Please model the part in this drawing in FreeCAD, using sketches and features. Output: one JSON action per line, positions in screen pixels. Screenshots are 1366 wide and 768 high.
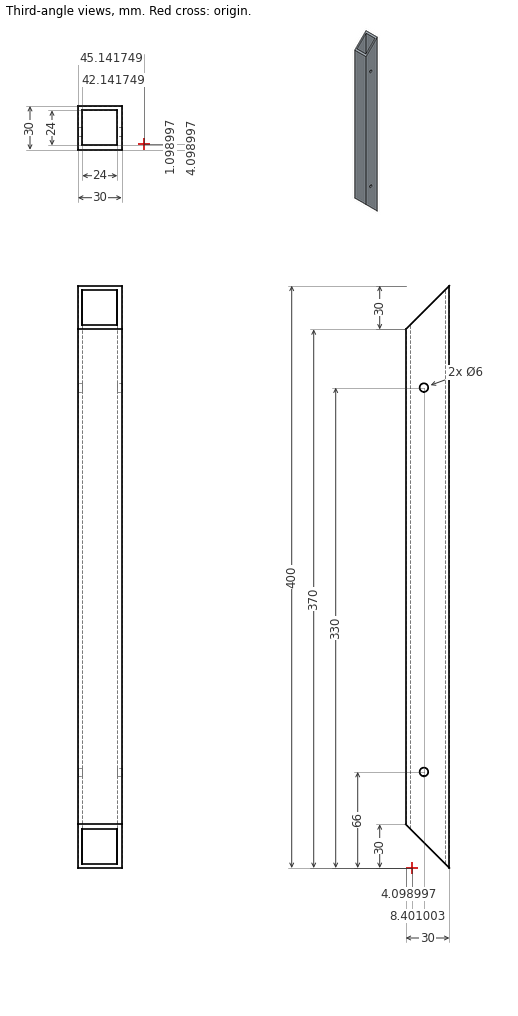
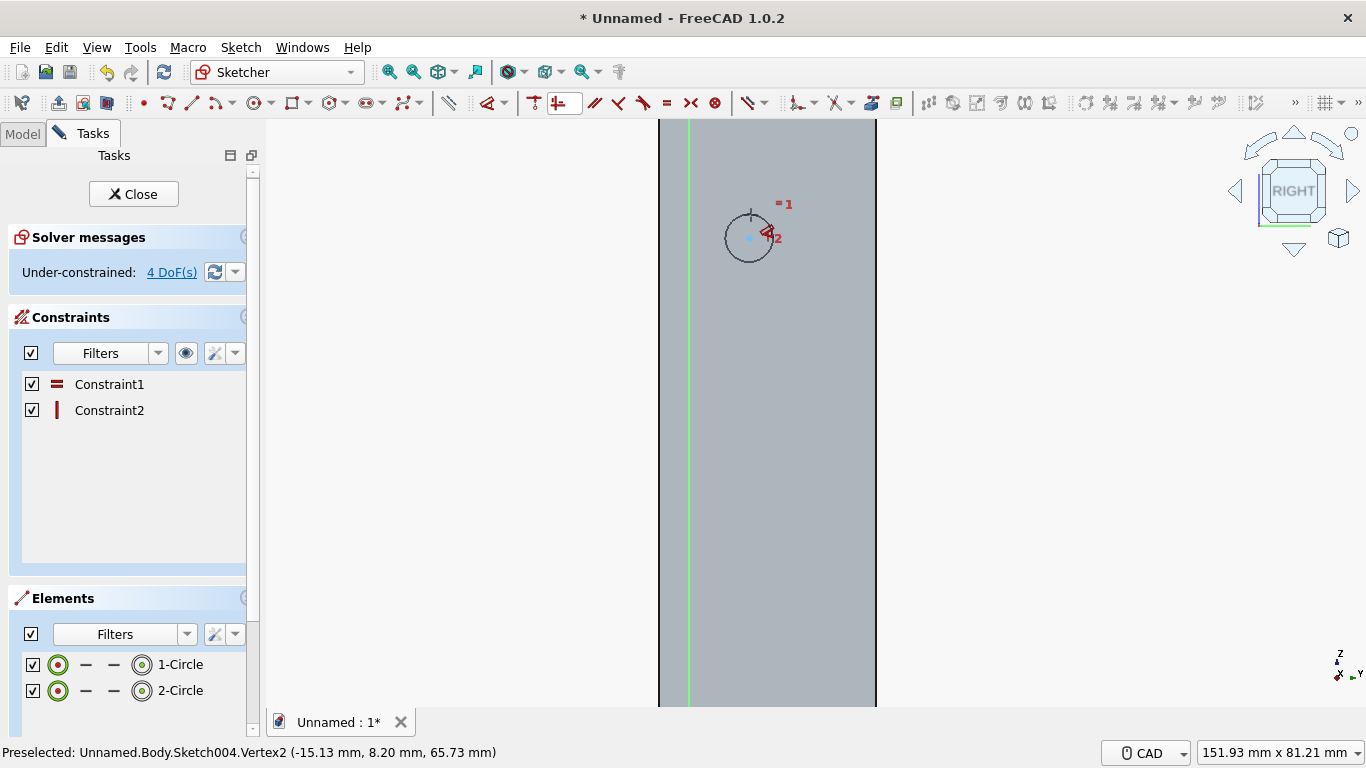
{"action": "left_click", "coordinate": [750, 214]}
{"action": "left_click", "coordinate": [751, 182]}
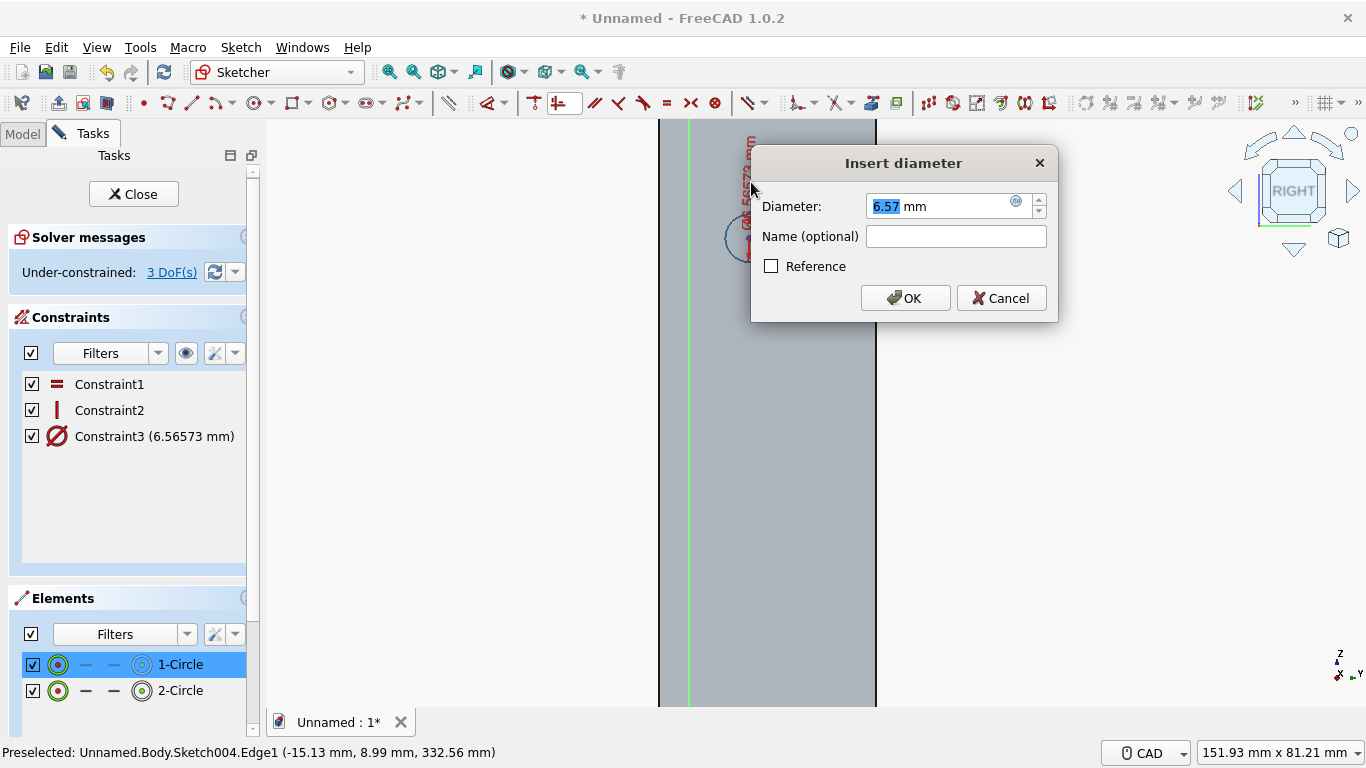
{"action": "type", "text": "6"}
{"action": "key", "text": "Return"}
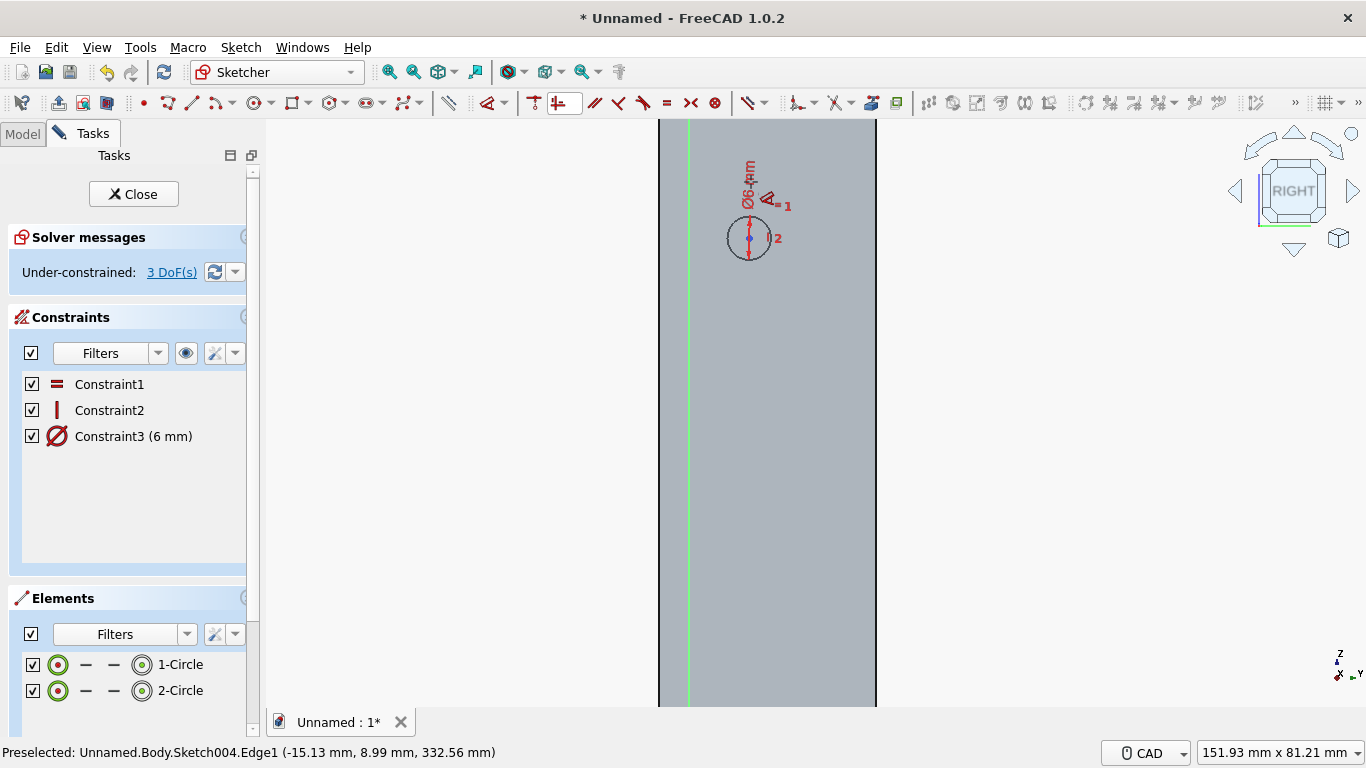
{"action": "scroll", "coordinate": [751, 214], "scroll_direction": "down", "scroll_amount": 9}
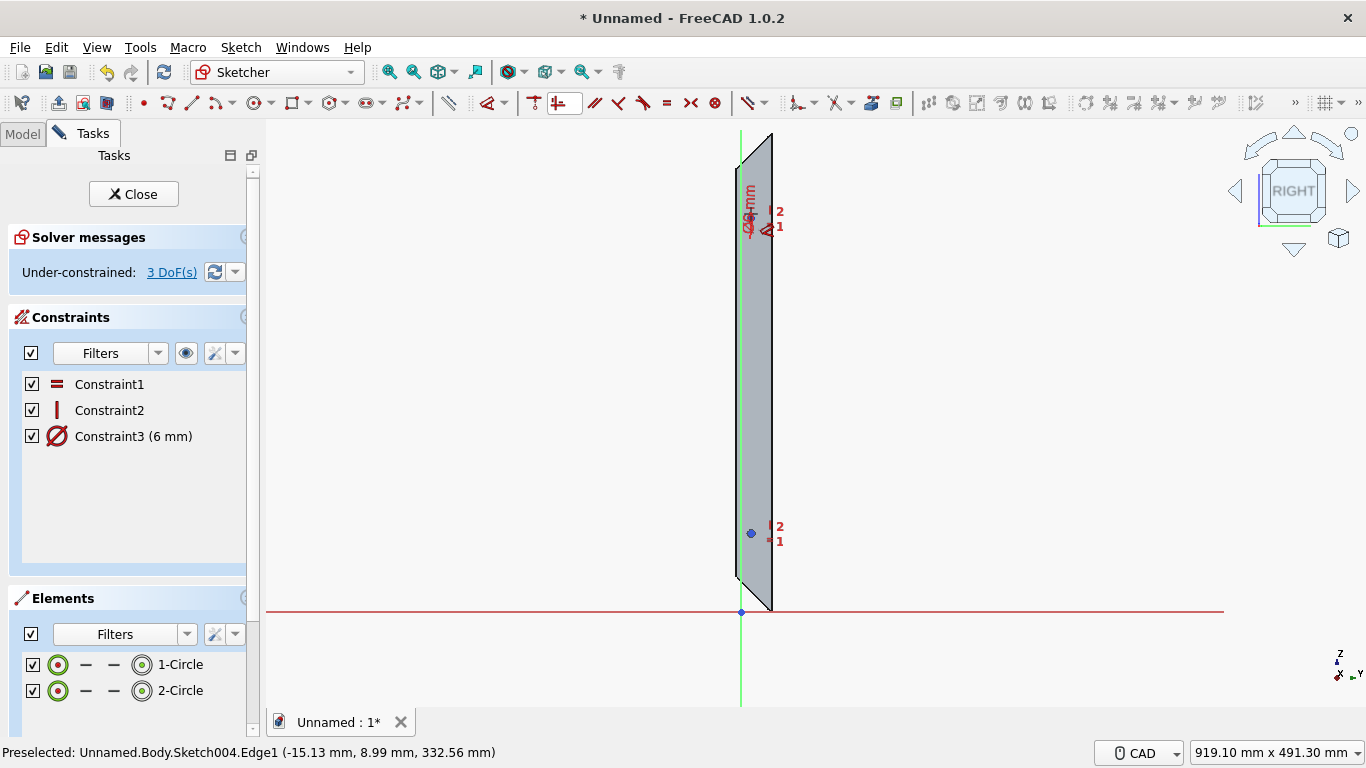
{"action": "left_click", "coordinate": [751, 534]}
{"action": "left_click", "coordinate": [707, 573]}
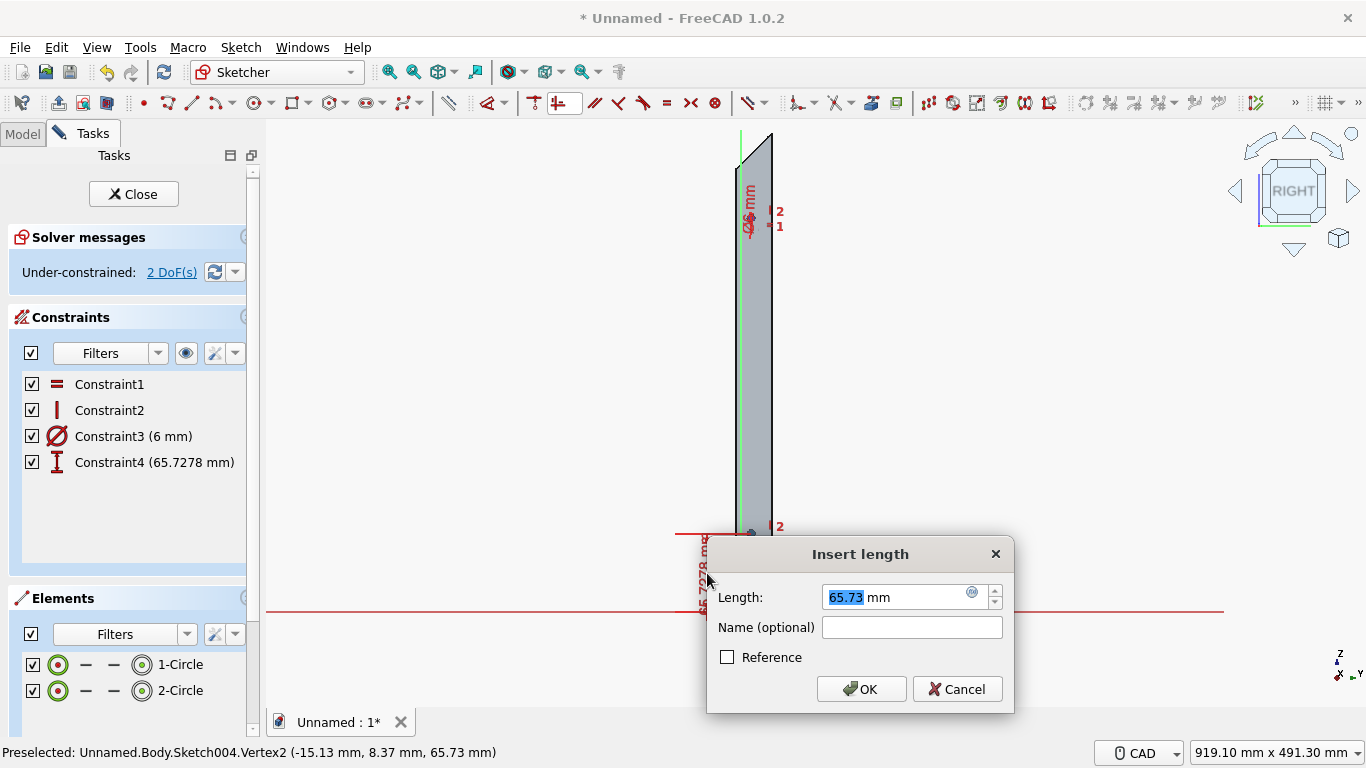
{"action": "type", "text": "66"}
{"action": "key", "text": "Return"}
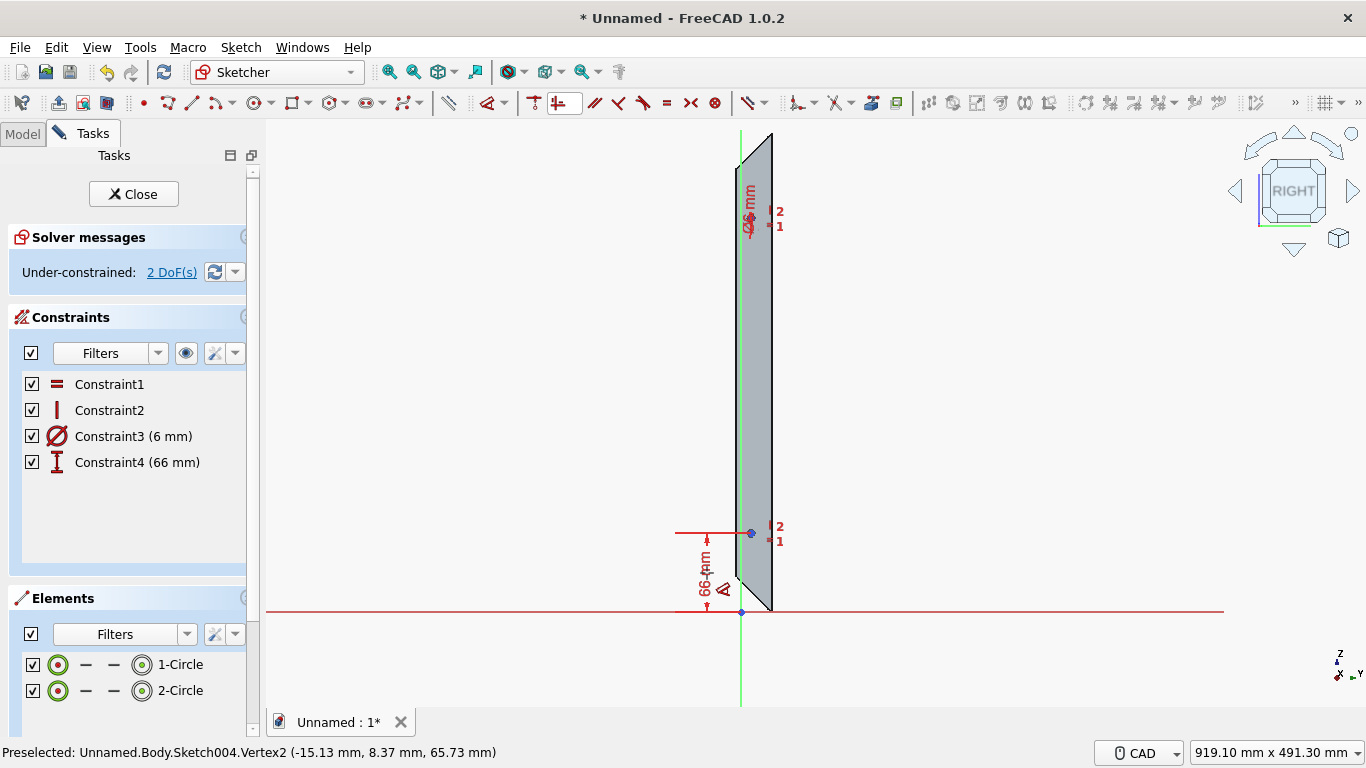
{"action": "left_click", "coordinate": [751, 218]}
{"action": "left_click", "coordinate": [707, 415]}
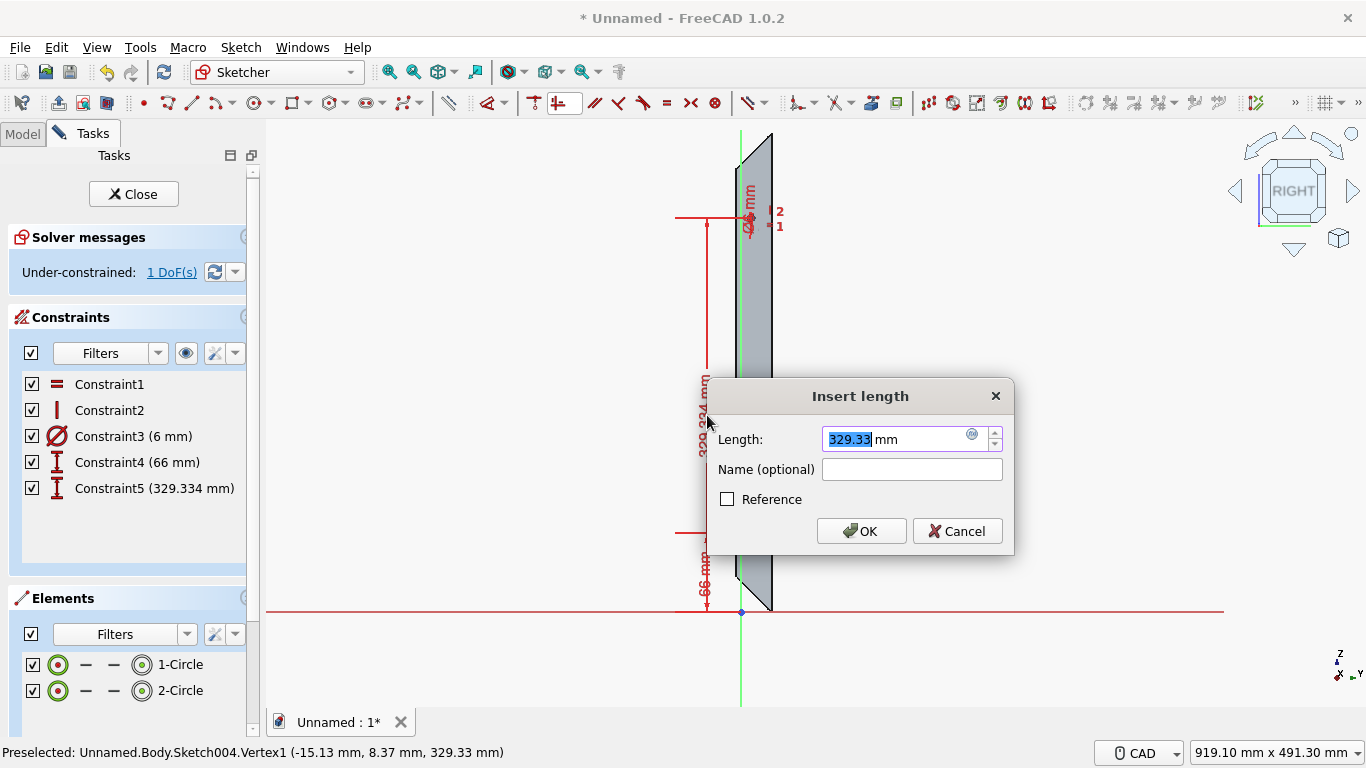
{"action": "type", "text": "330"}
{"action": "key", "text": "Return"}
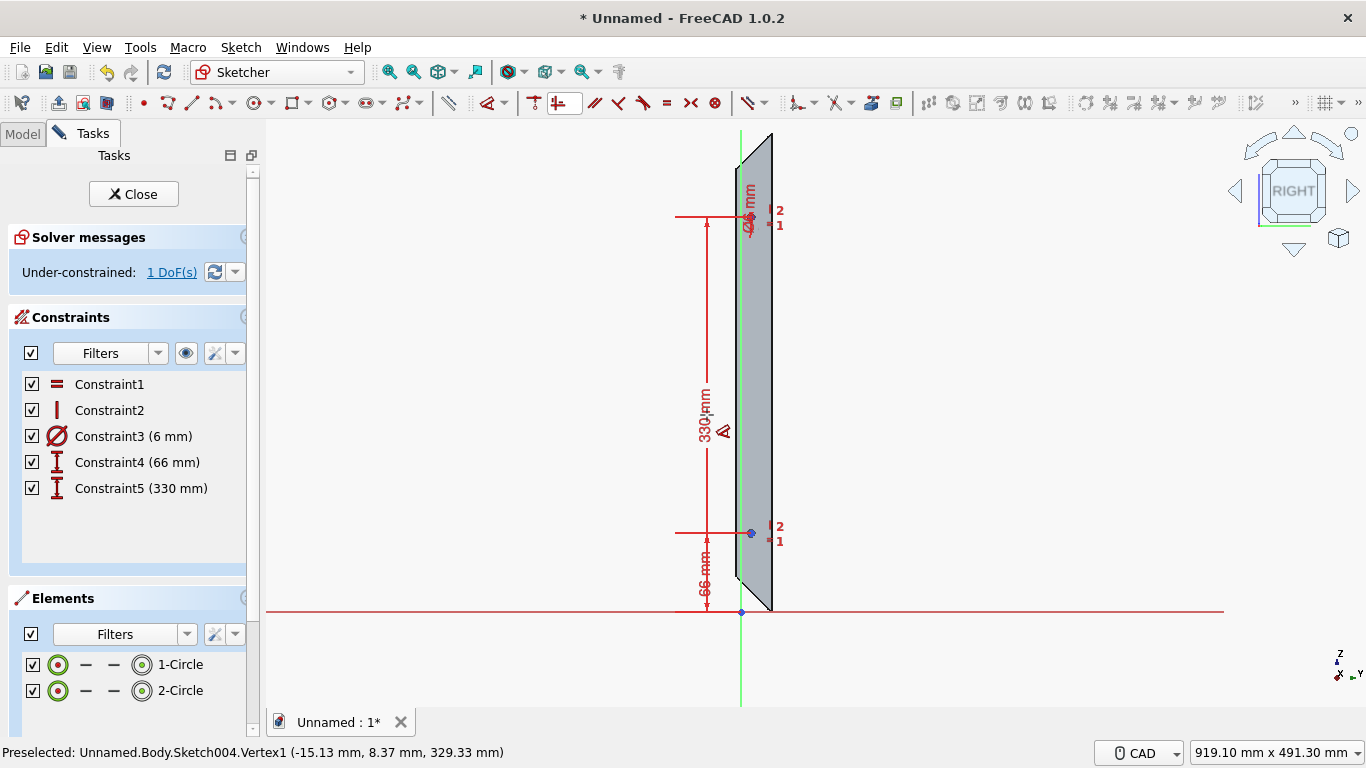
{"action": "scroll", "coordinate": [751, 217], "scroll_direction": "up", "scroll_amount": 7}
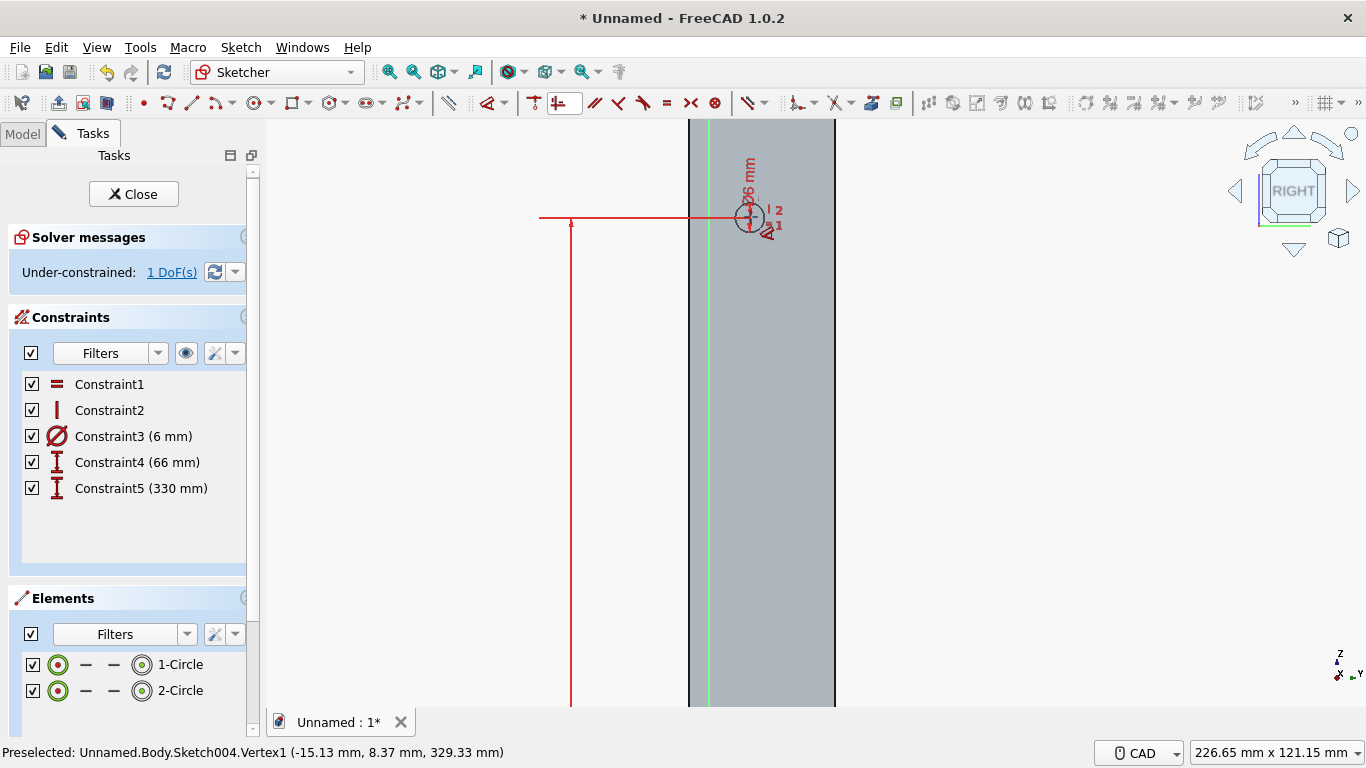
{"action": "left_click", "coordinate": [750, 218]}
{"action": "left_click", "coordinate": [730, 160]}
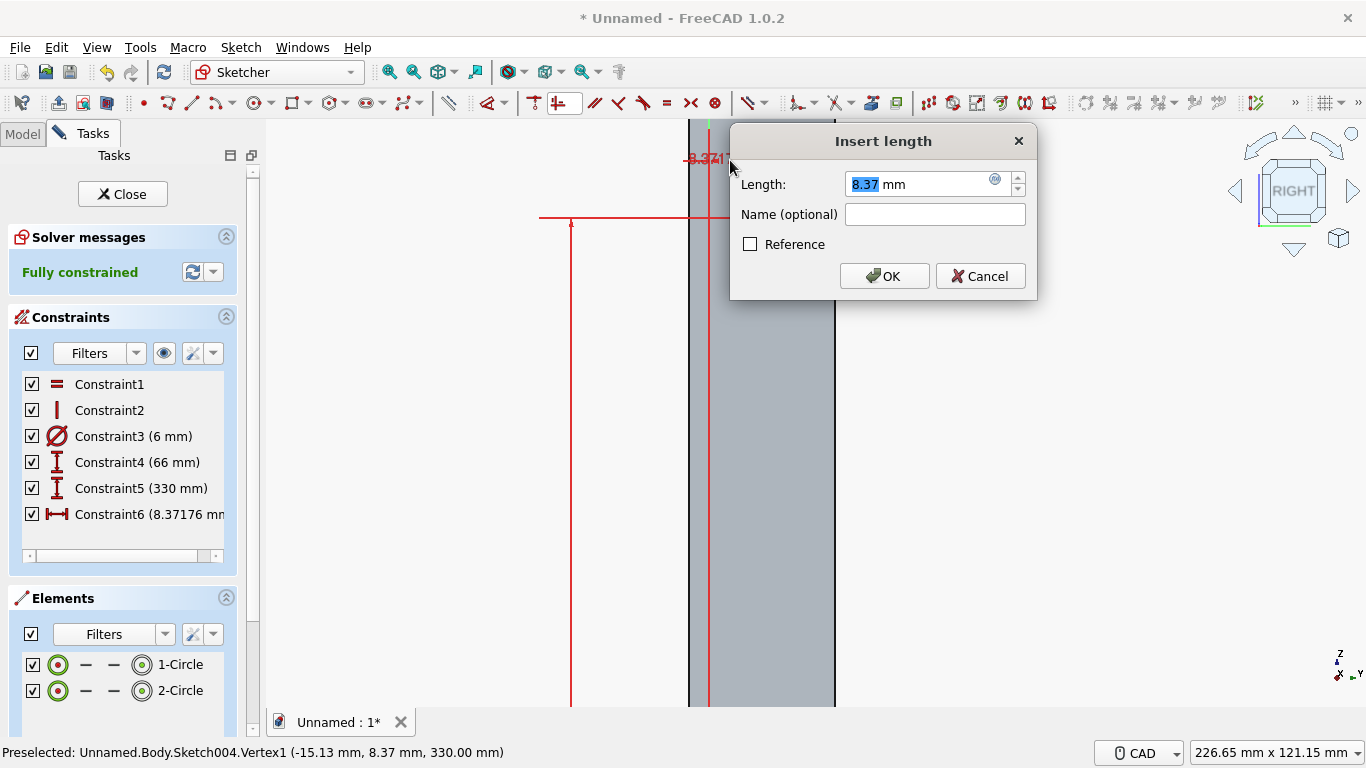
{"action": "type", "text": "8.401003"}
{"action": "key", "text": "Return"}
{"action": "key", "text": "Escape"}